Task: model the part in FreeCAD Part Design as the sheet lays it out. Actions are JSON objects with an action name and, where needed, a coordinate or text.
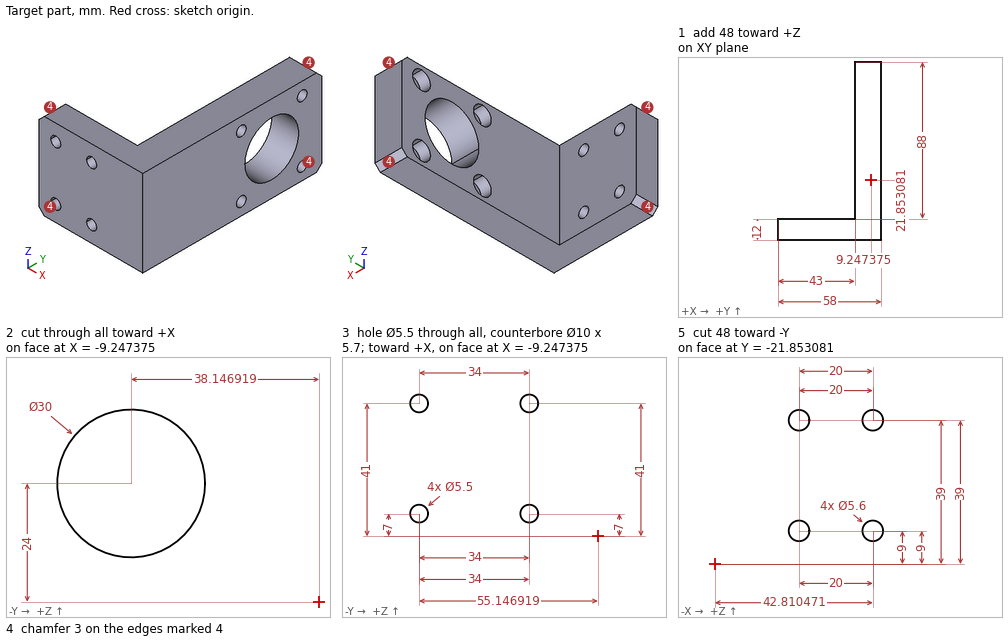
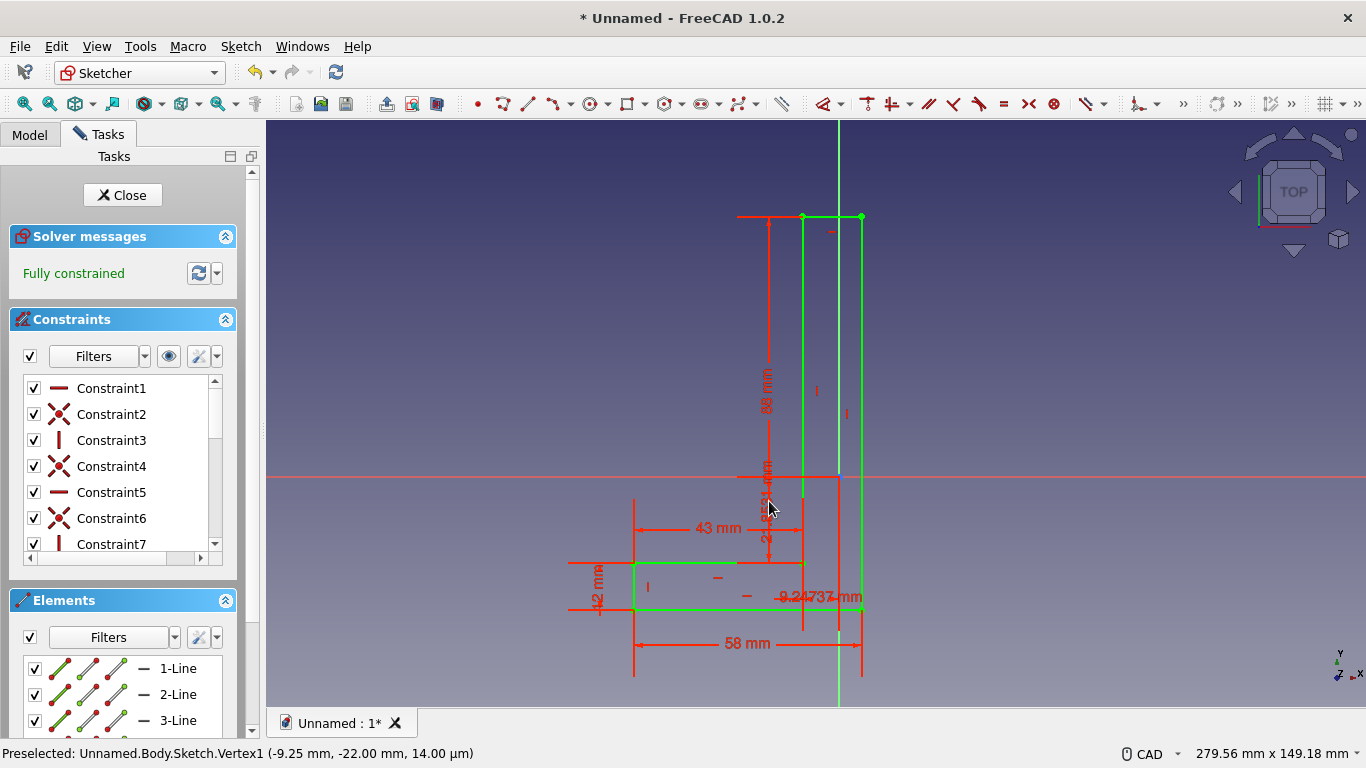
{"action": "left_click", "coordinate": [123, 195]}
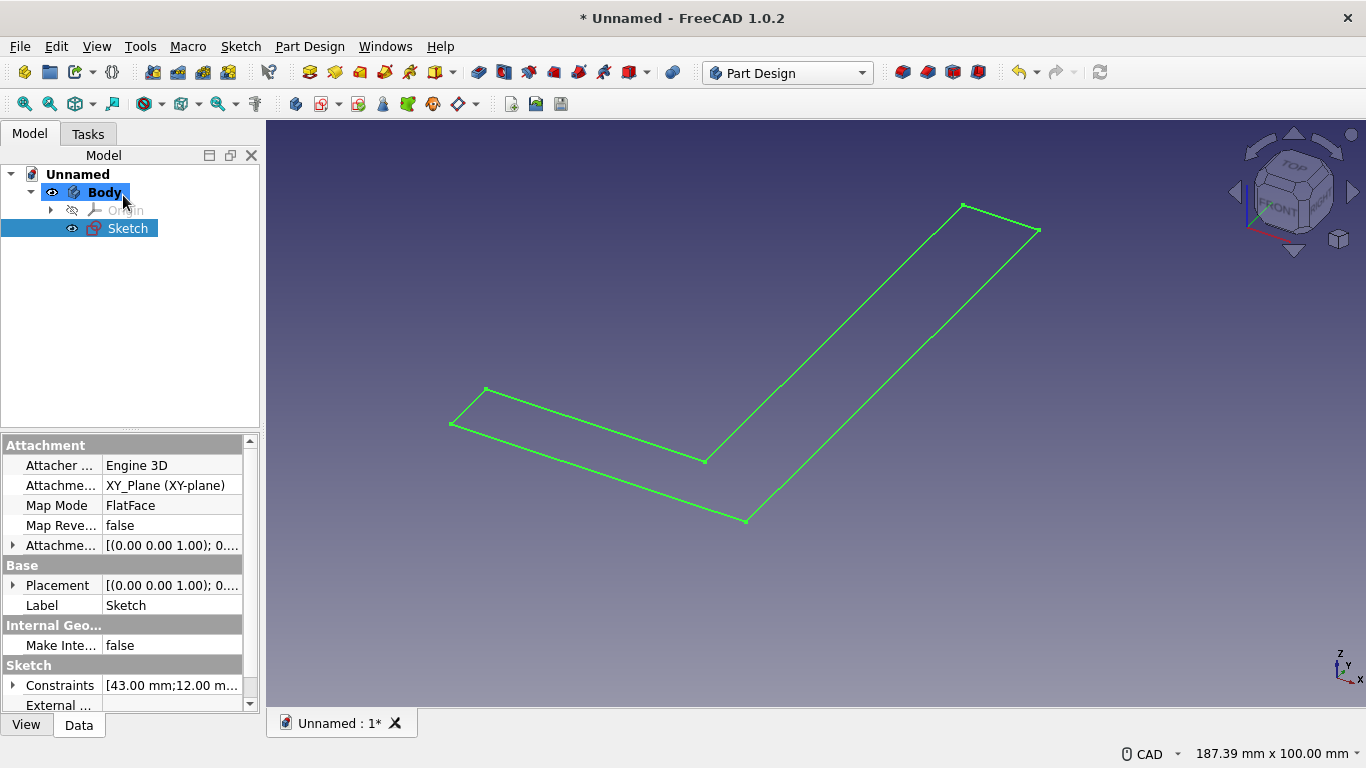
{"action": "left_click", "coordinate": [310, 72]}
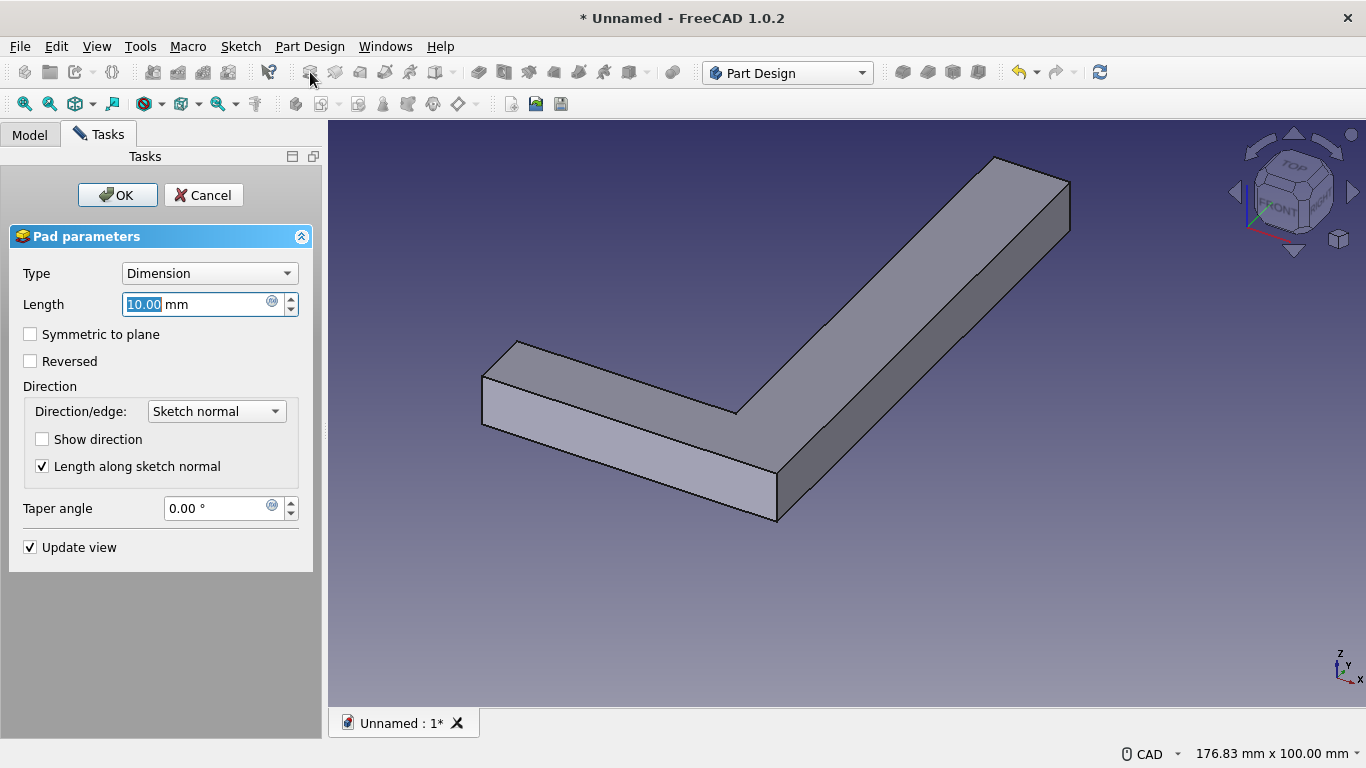
{"action": "type", "text": "48"}
{"action": "key", "text": "Tab"}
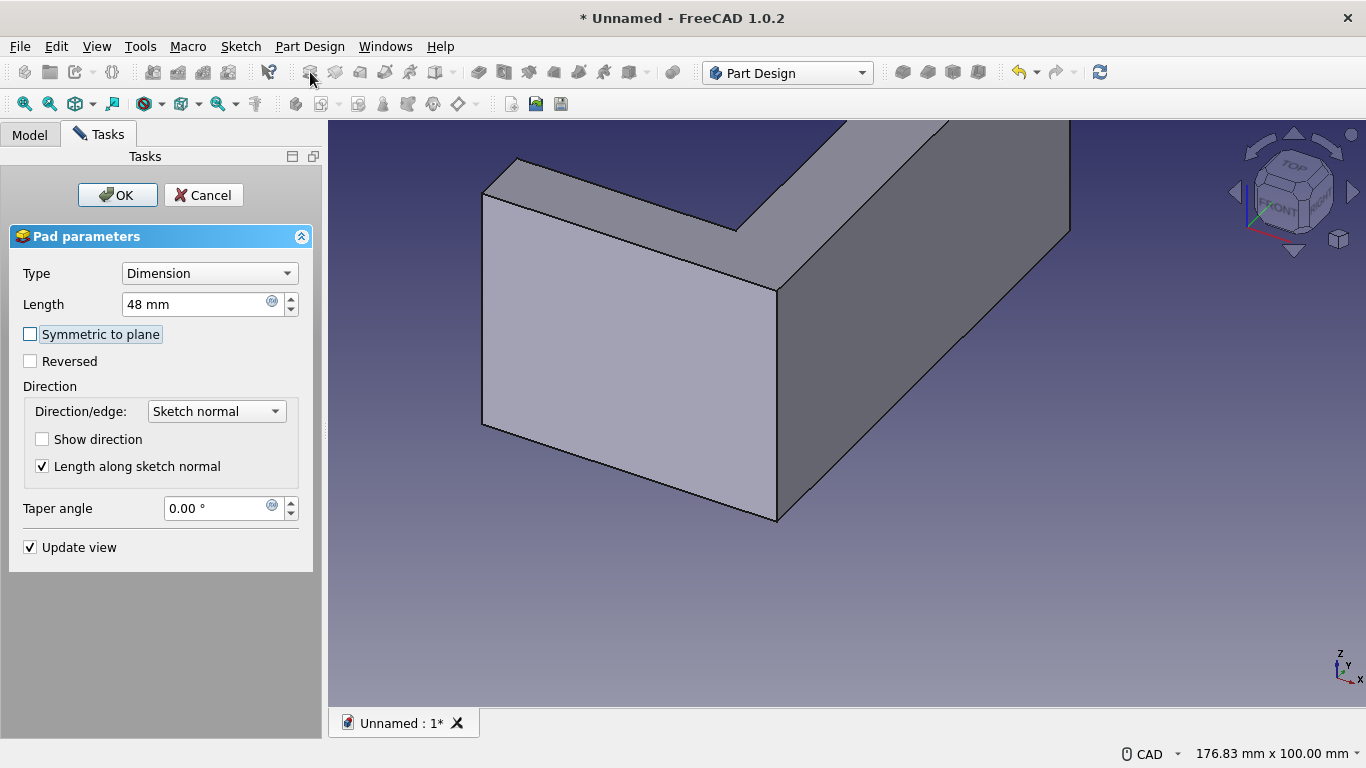
{"action": "left_click", "coordinate": [118, 195]}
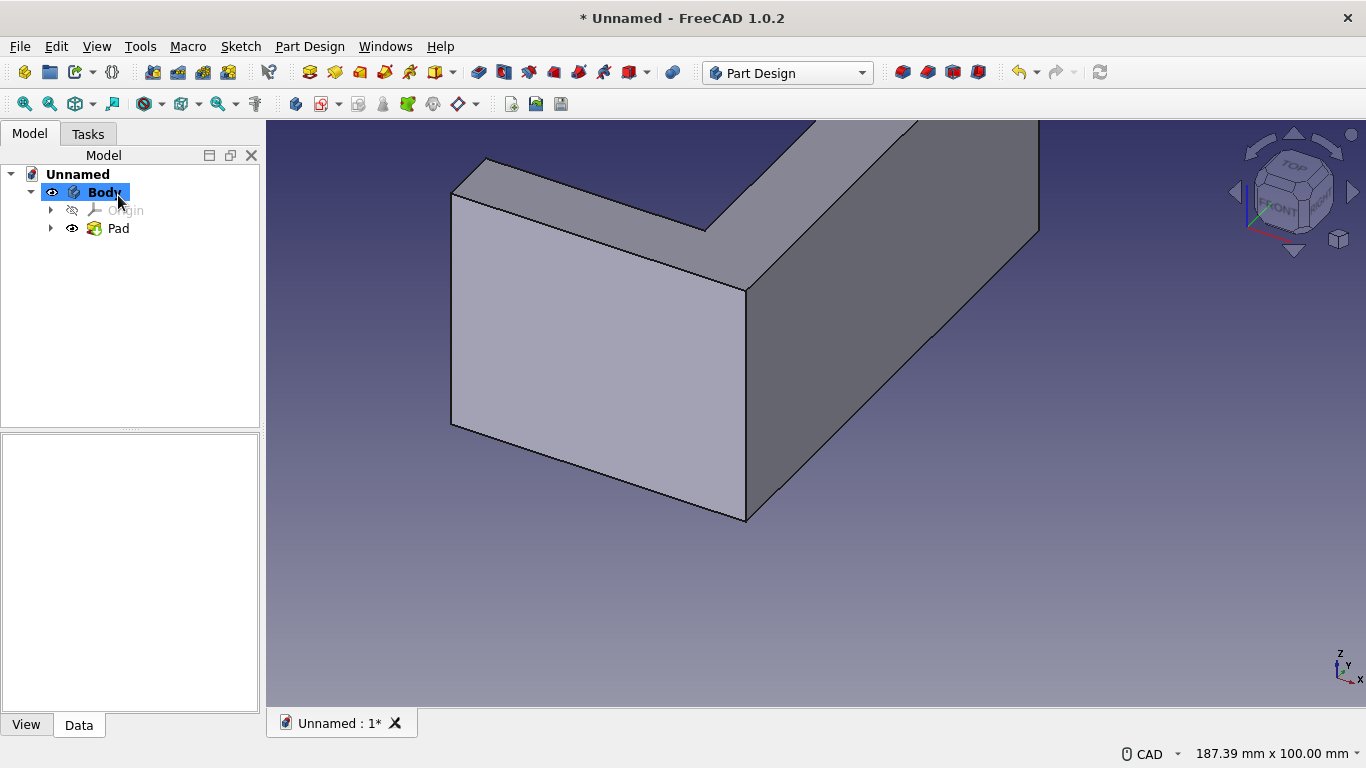
{"action": "left_click", "coordinate": [25, 104]}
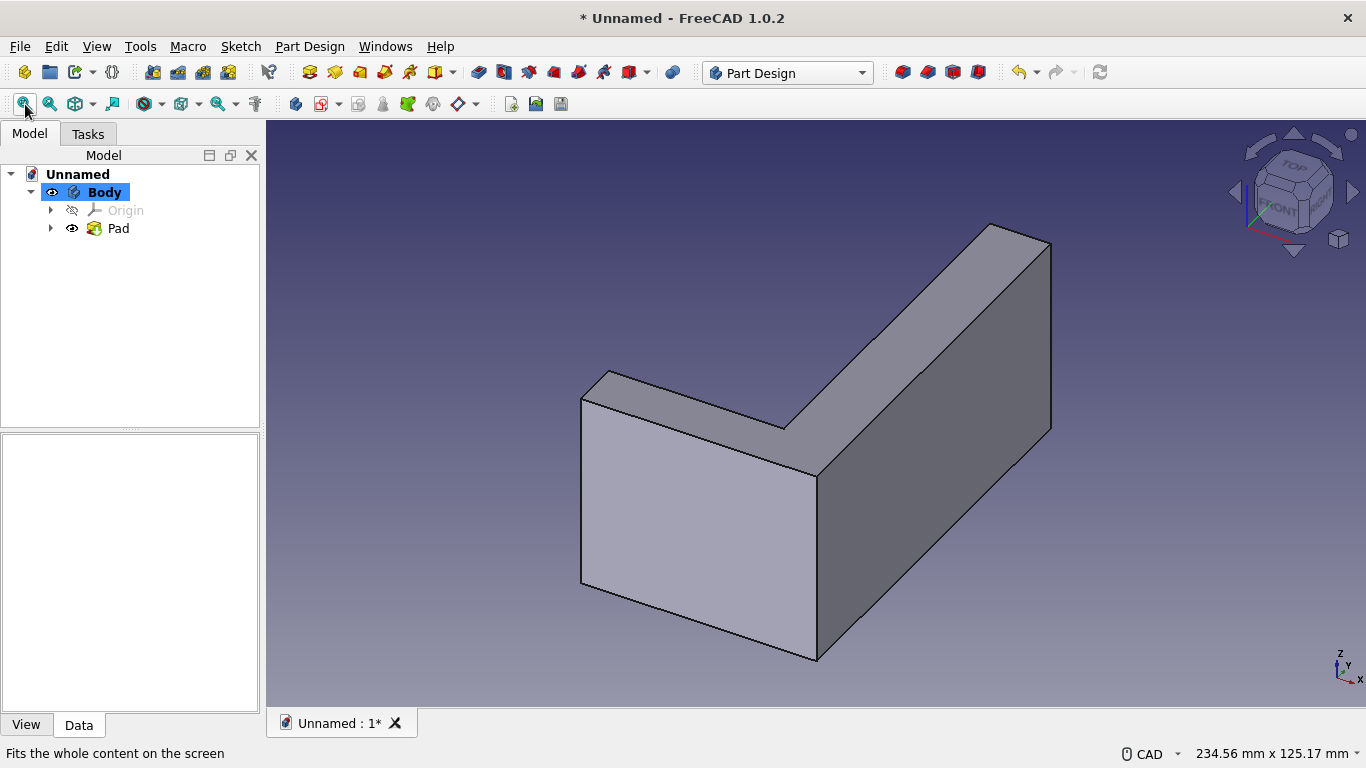
{"action": "key", "text": "6"}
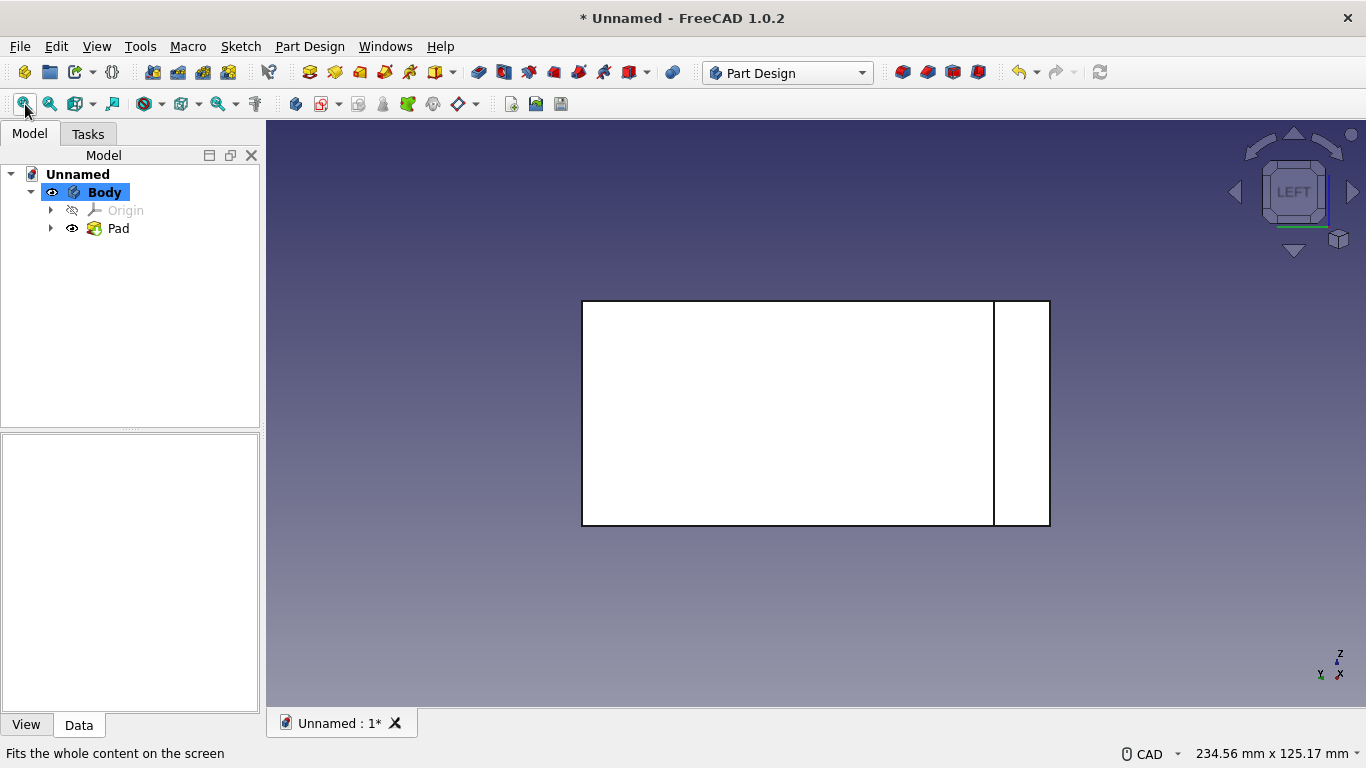
{"action": "left_click", "coordinate": [25, 104]}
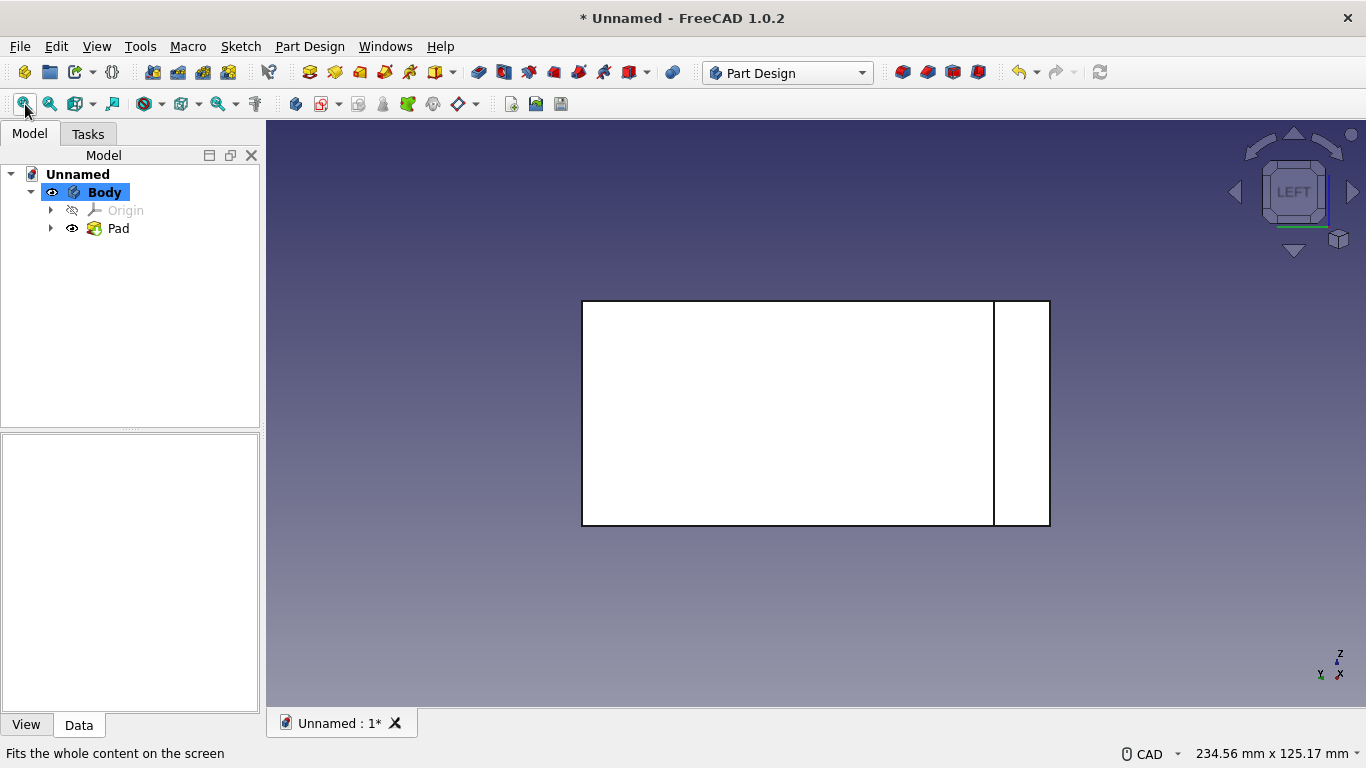
{"action": "left_click", "coordinate": [729, 412]}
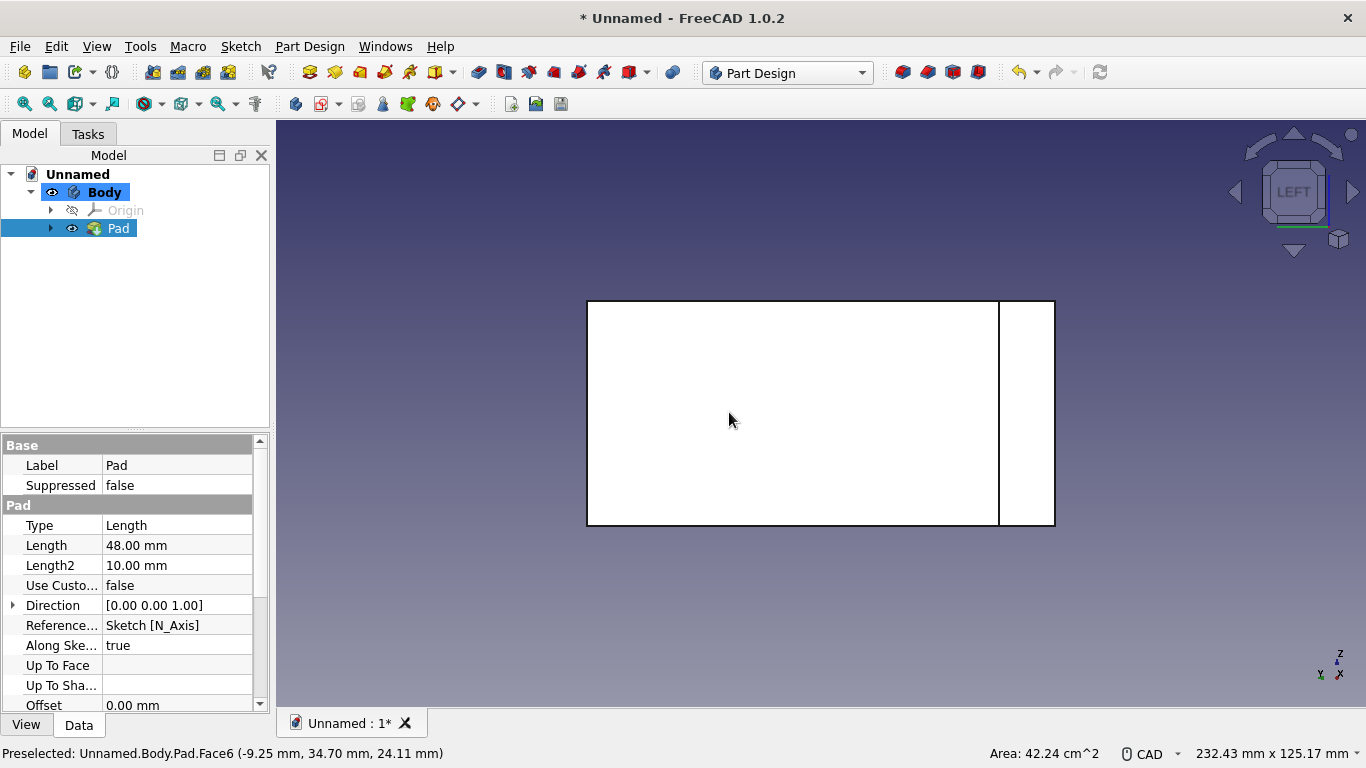
{"action": "left_click", "coordinate": [320, 104]}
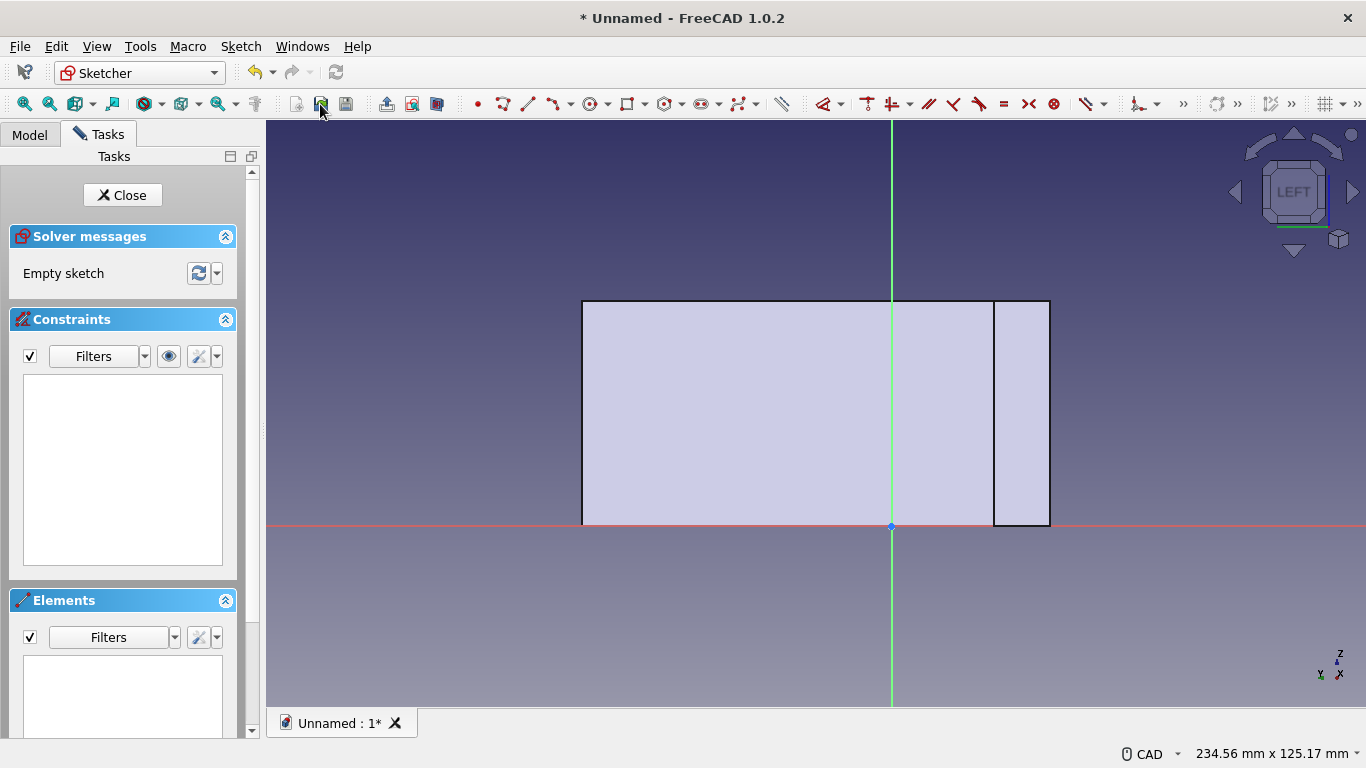
{"action": "key", "text": "q s"}